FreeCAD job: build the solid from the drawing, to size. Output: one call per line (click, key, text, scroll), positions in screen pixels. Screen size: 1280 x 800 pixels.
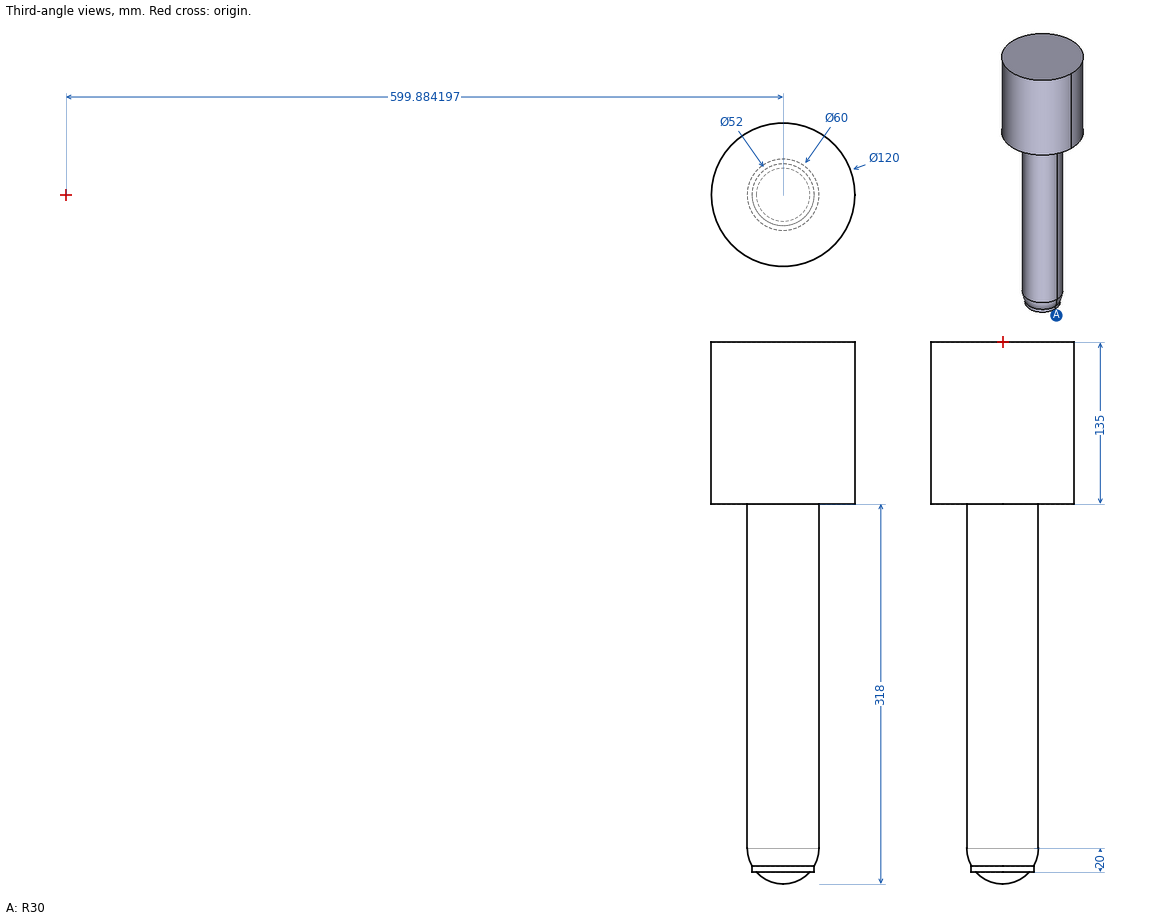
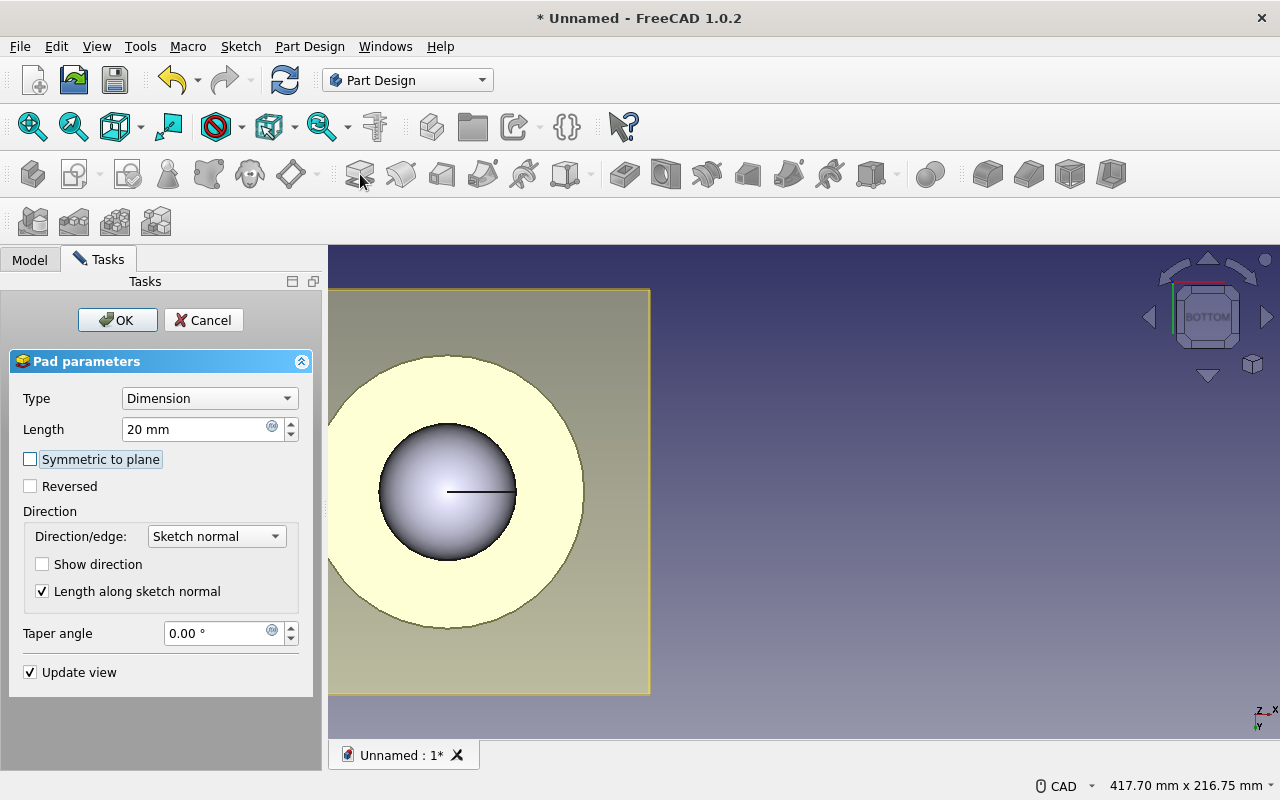
click(31, 486)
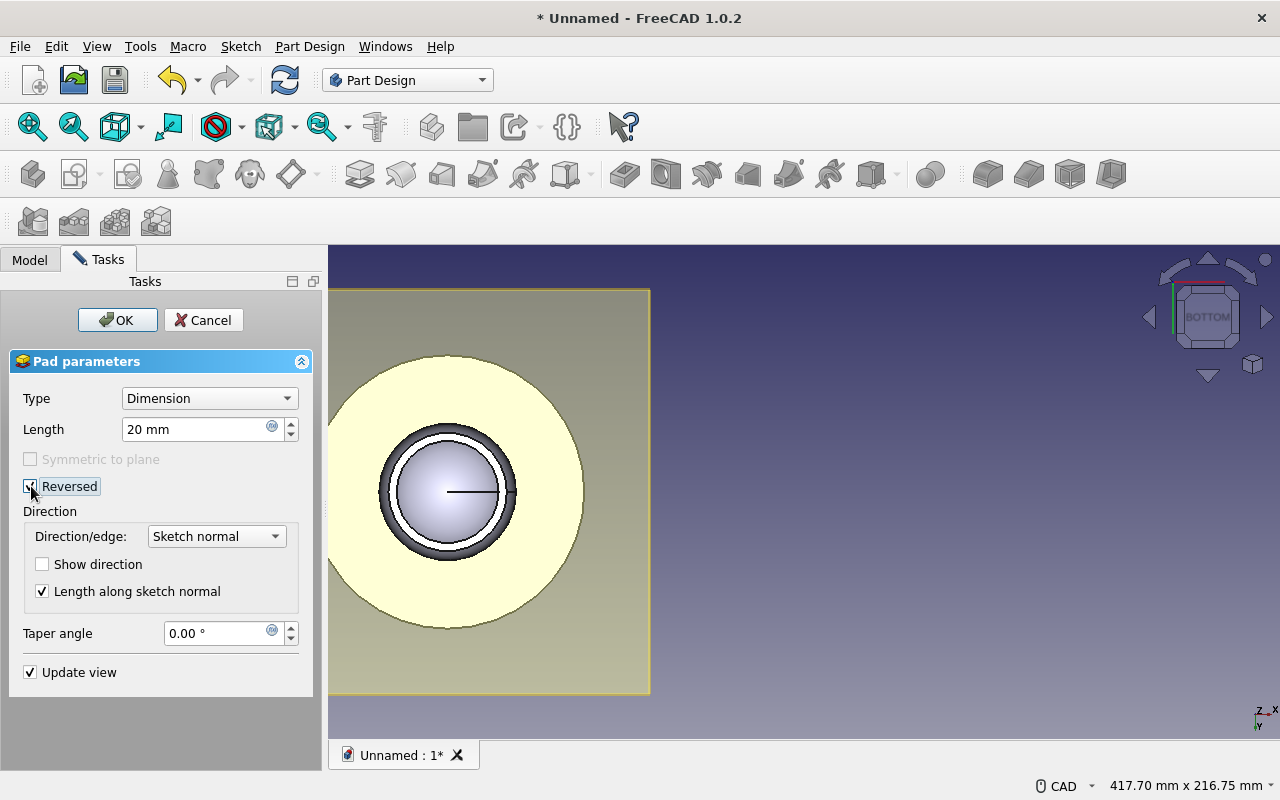
click(118, 320)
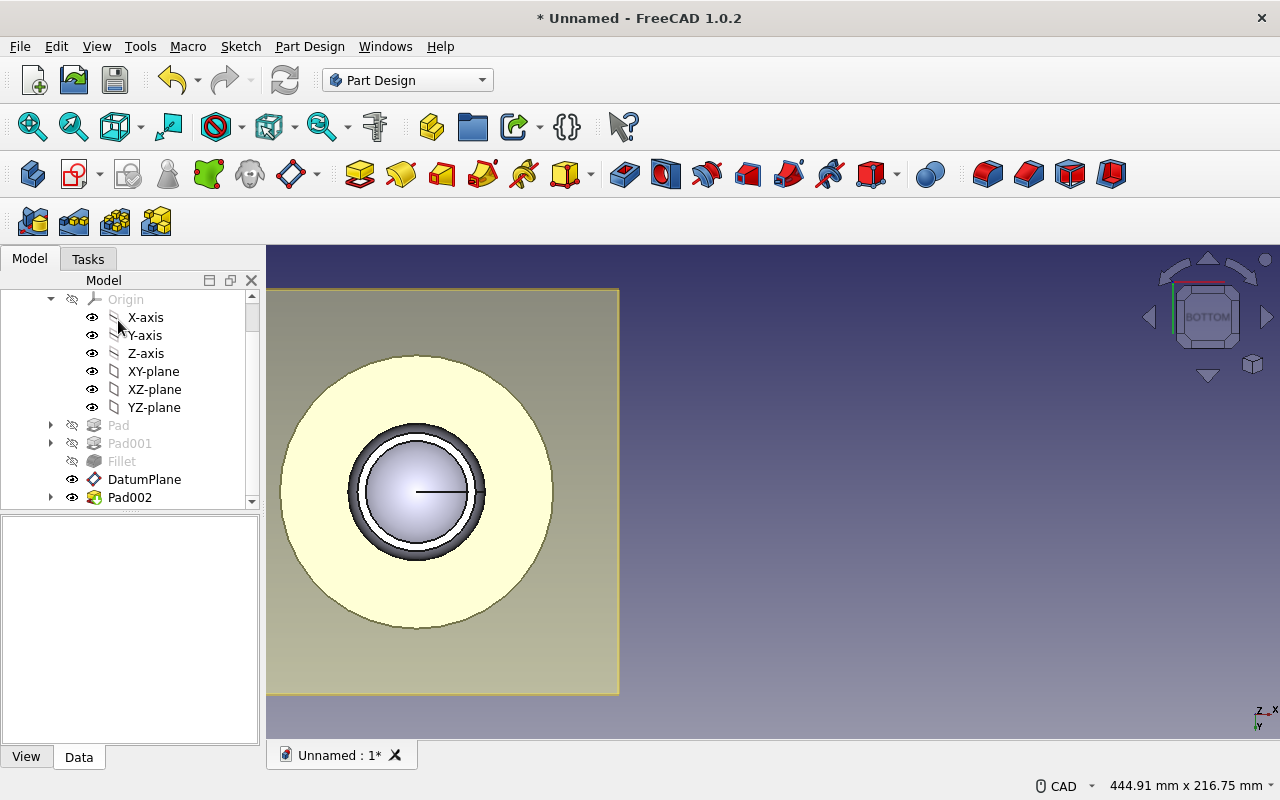
click(117, 479)
key(space)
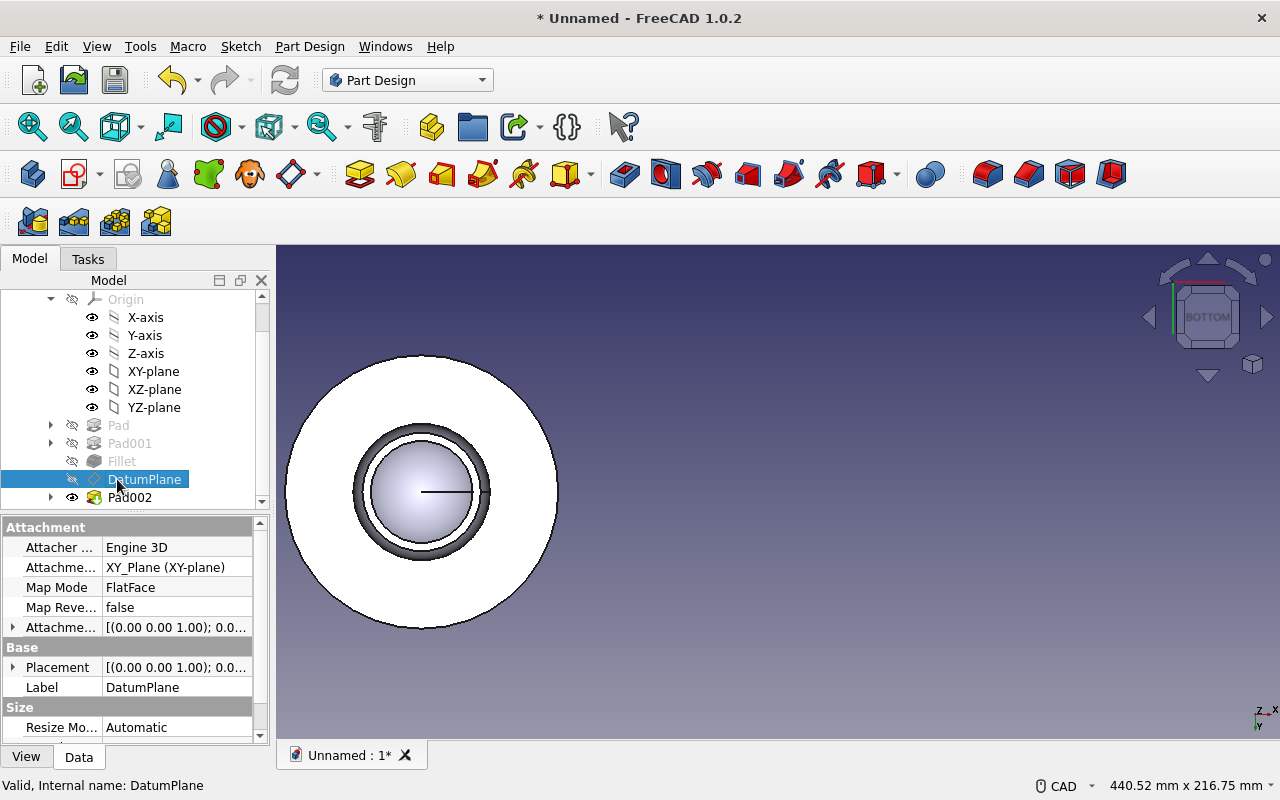
key(0)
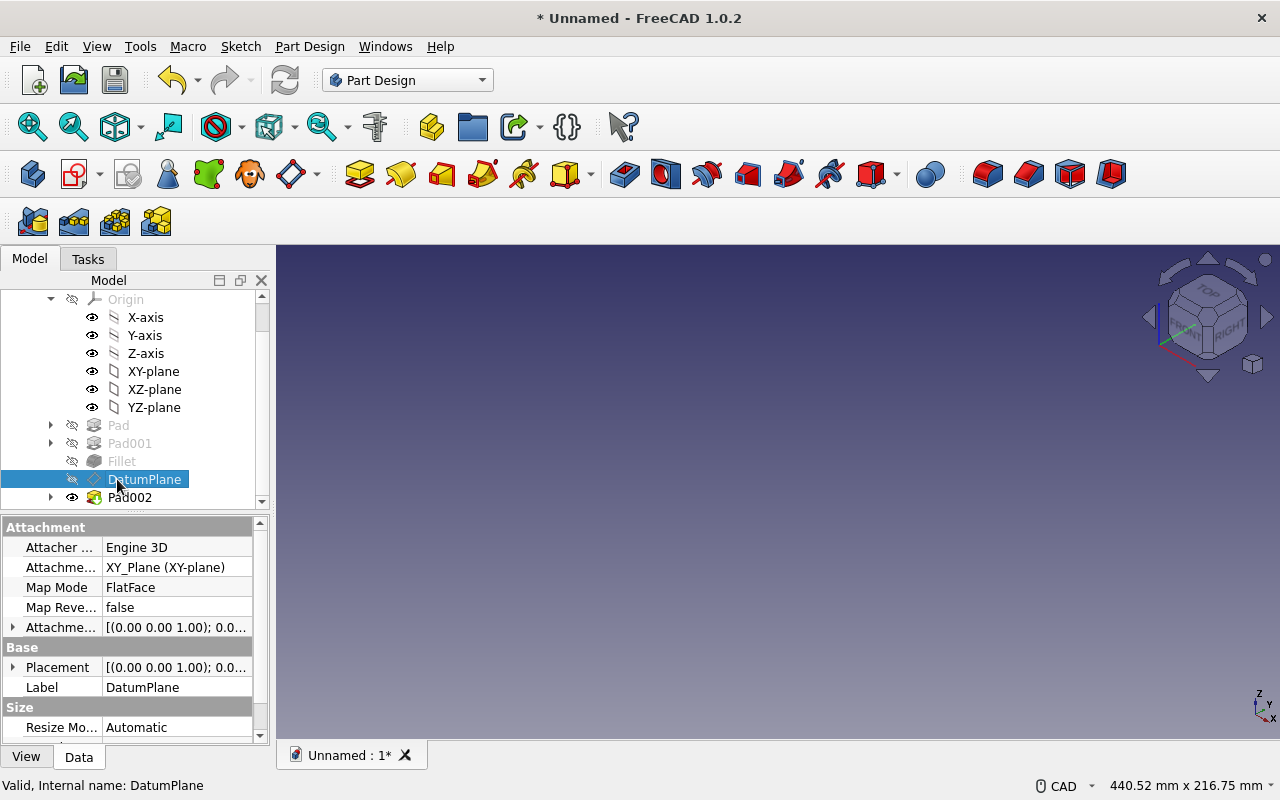
click(33, 128)